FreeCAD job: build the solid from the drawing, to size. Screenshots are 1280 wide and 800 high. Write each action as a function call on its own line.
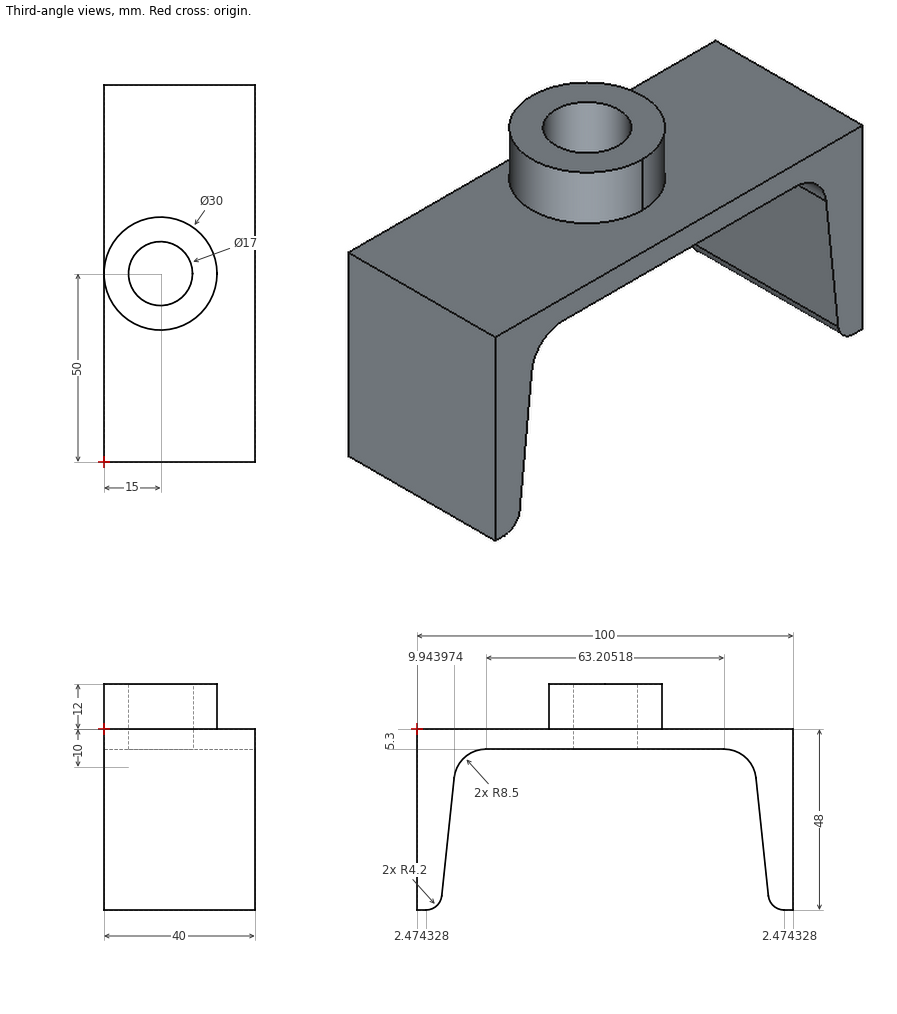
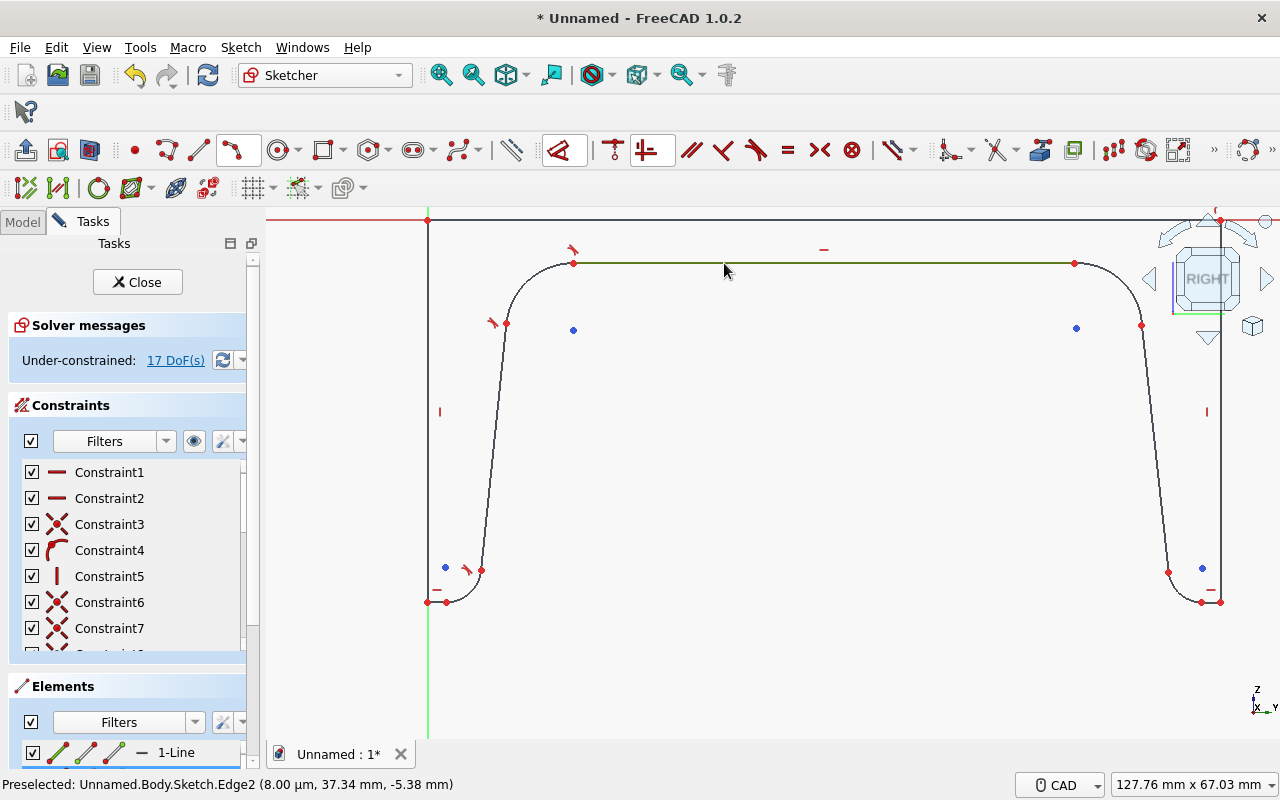
click(1104, 269)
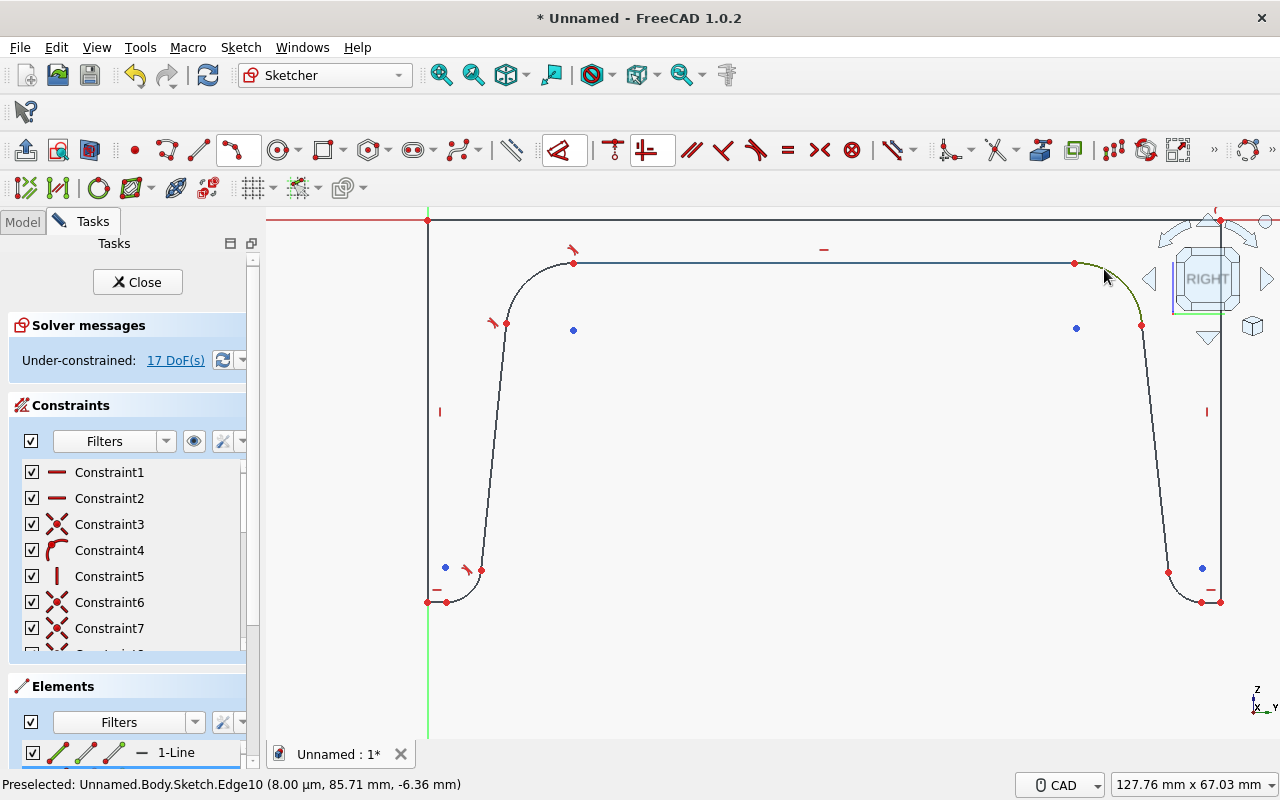
click(756, 150)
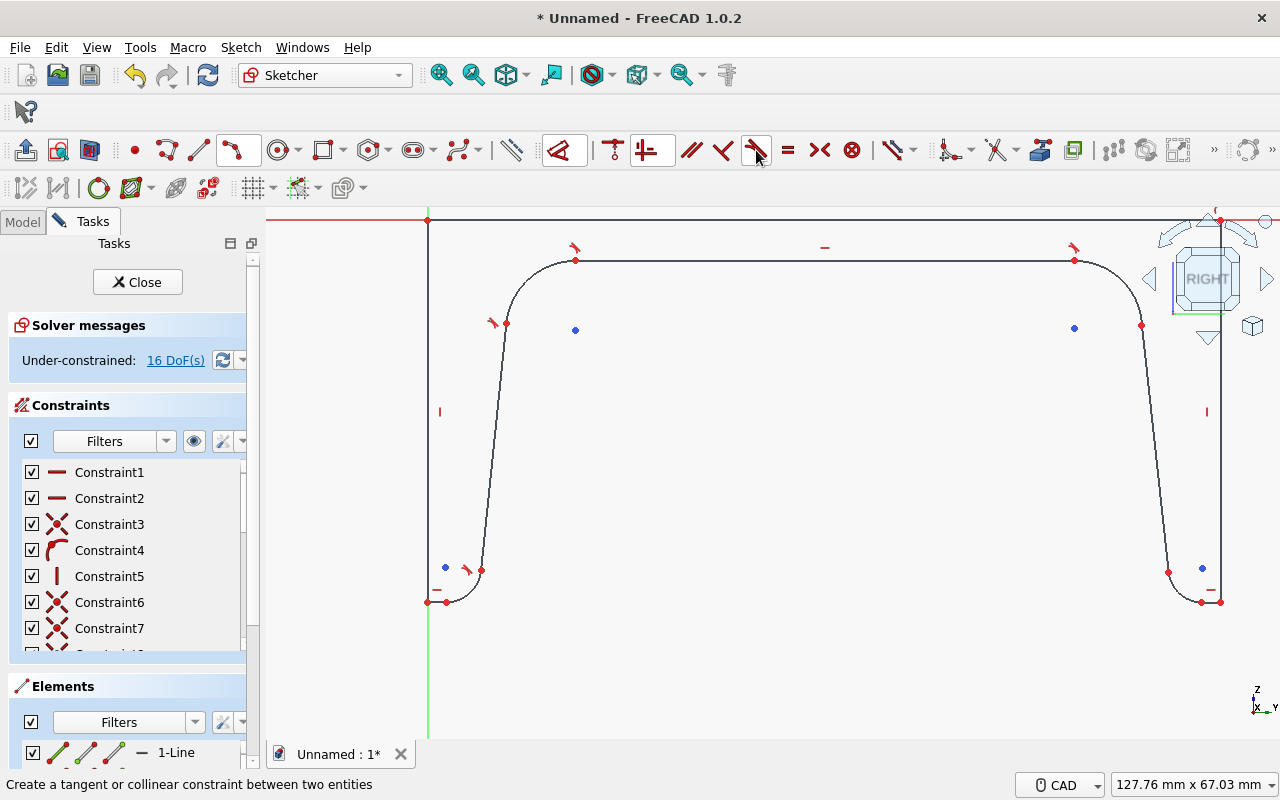
scroll(461, 599, down, 2)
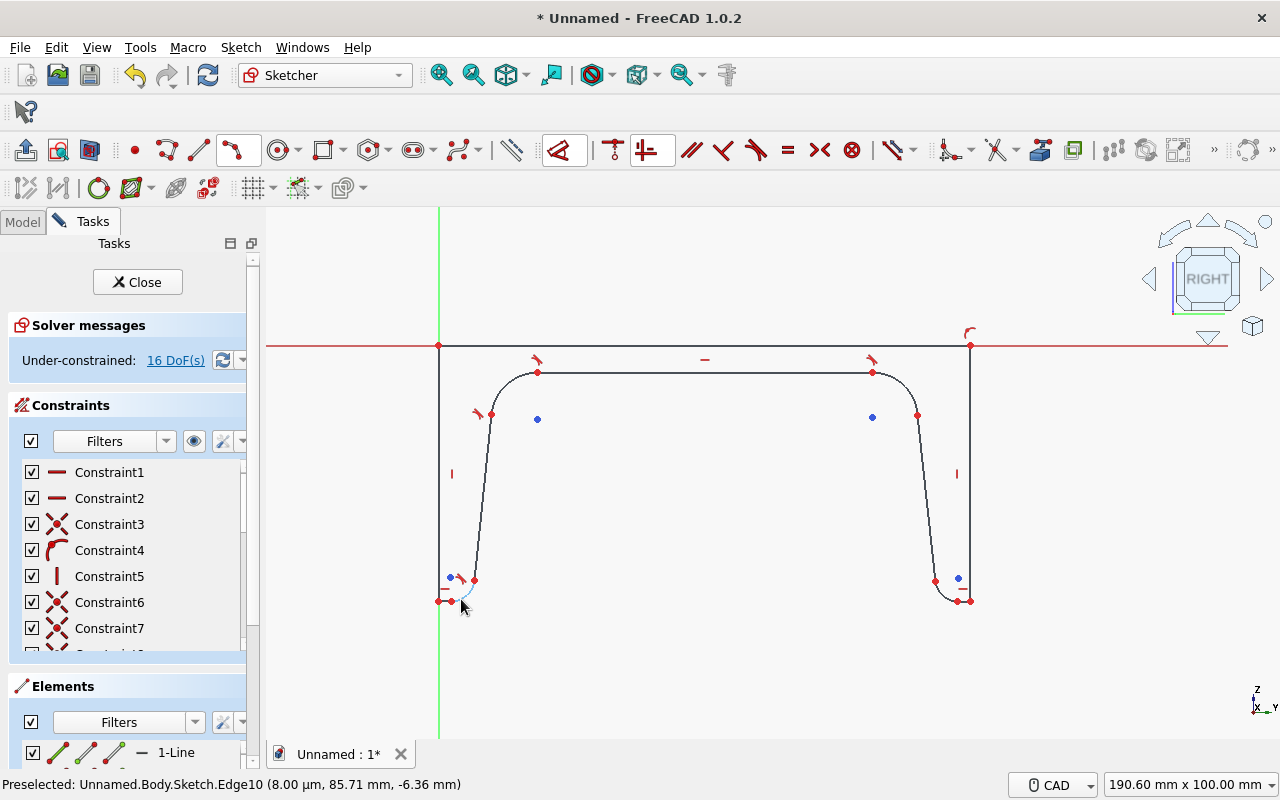
click(923, 465)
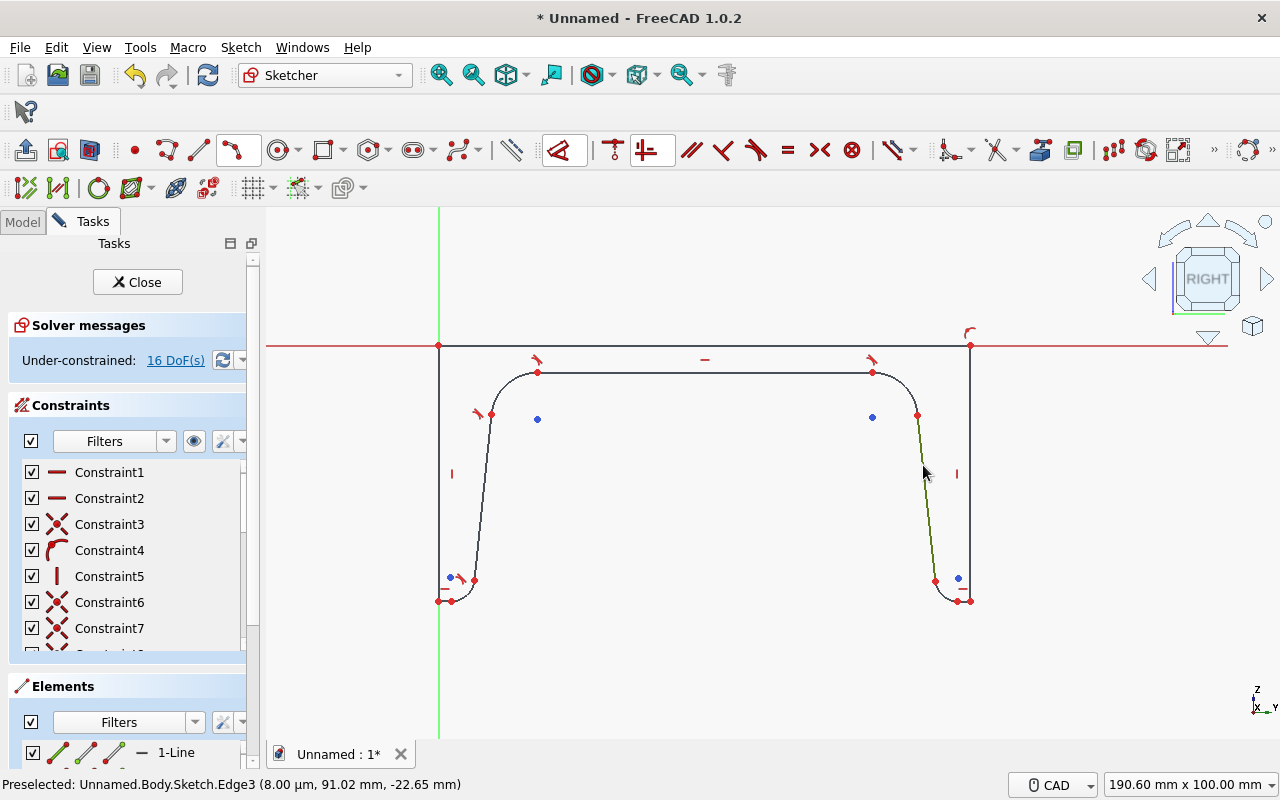
click(912, 396)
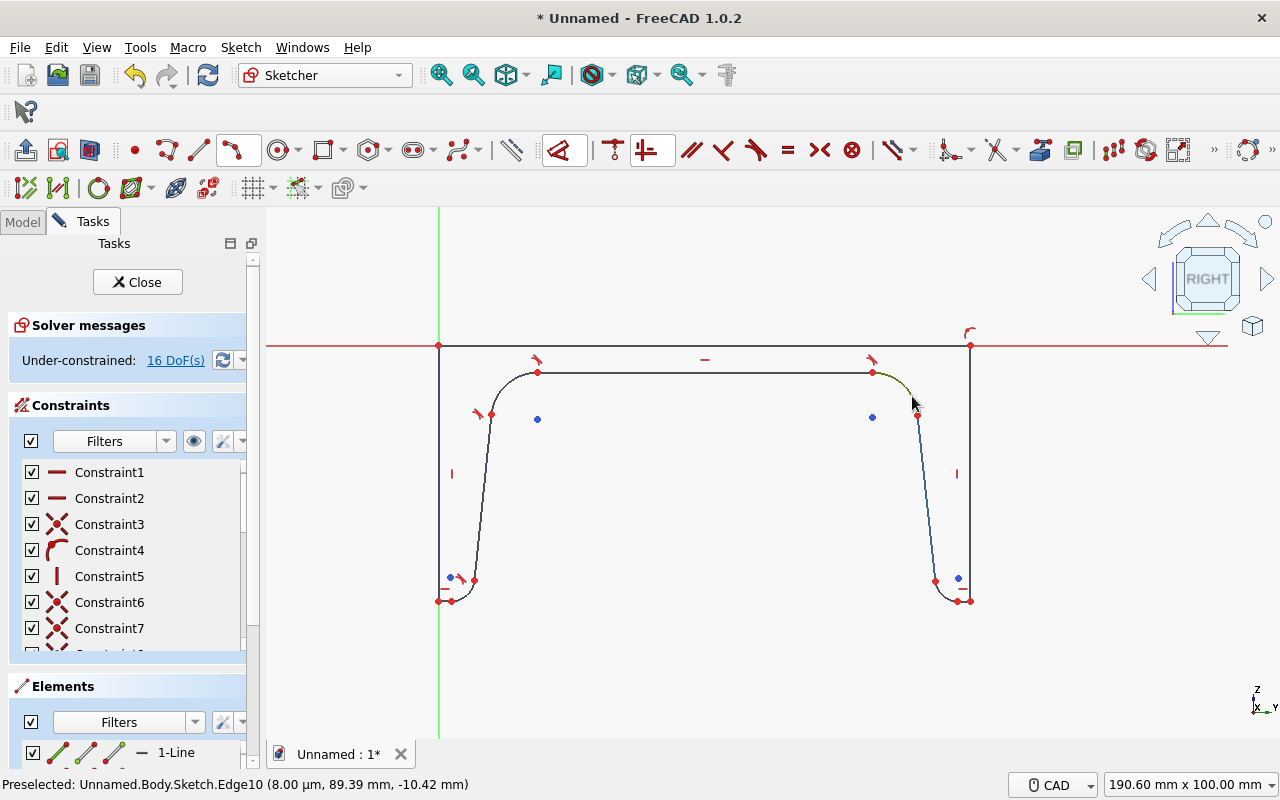
click(756, 150)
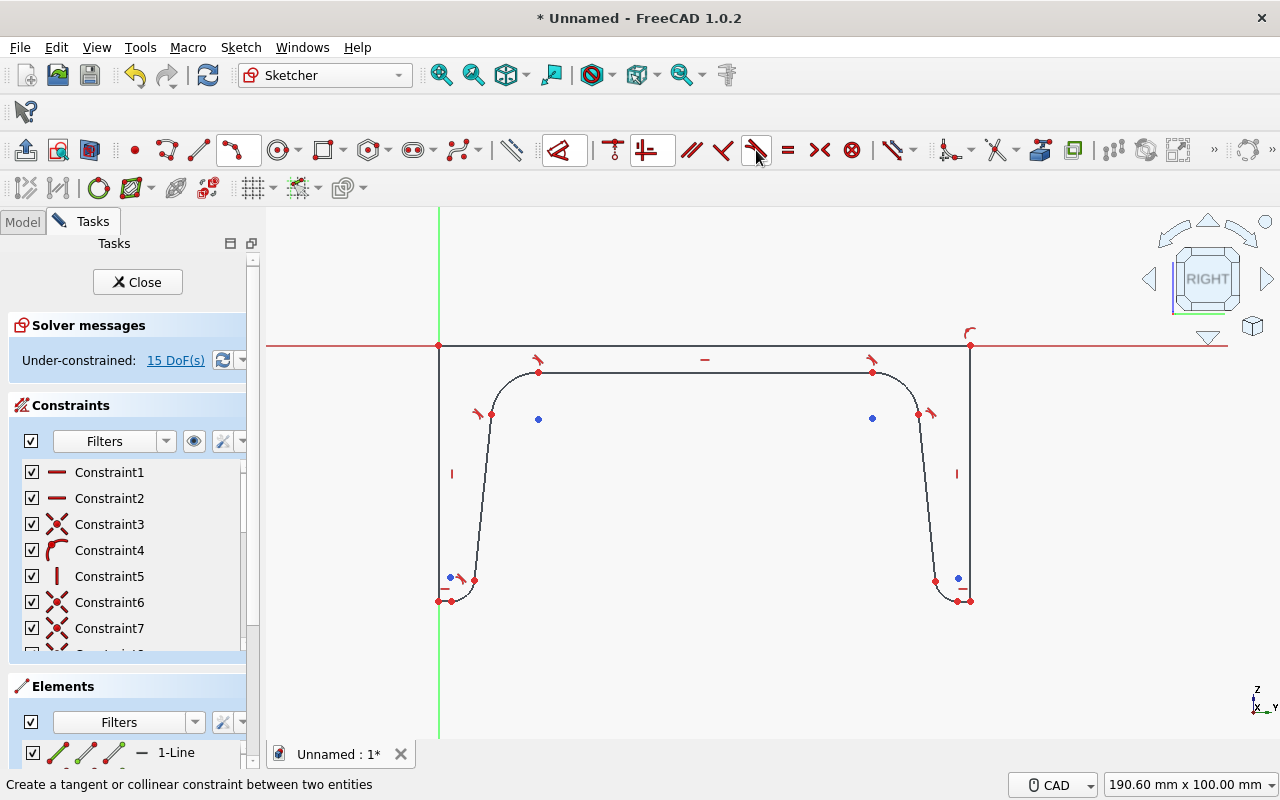
click(924, 465)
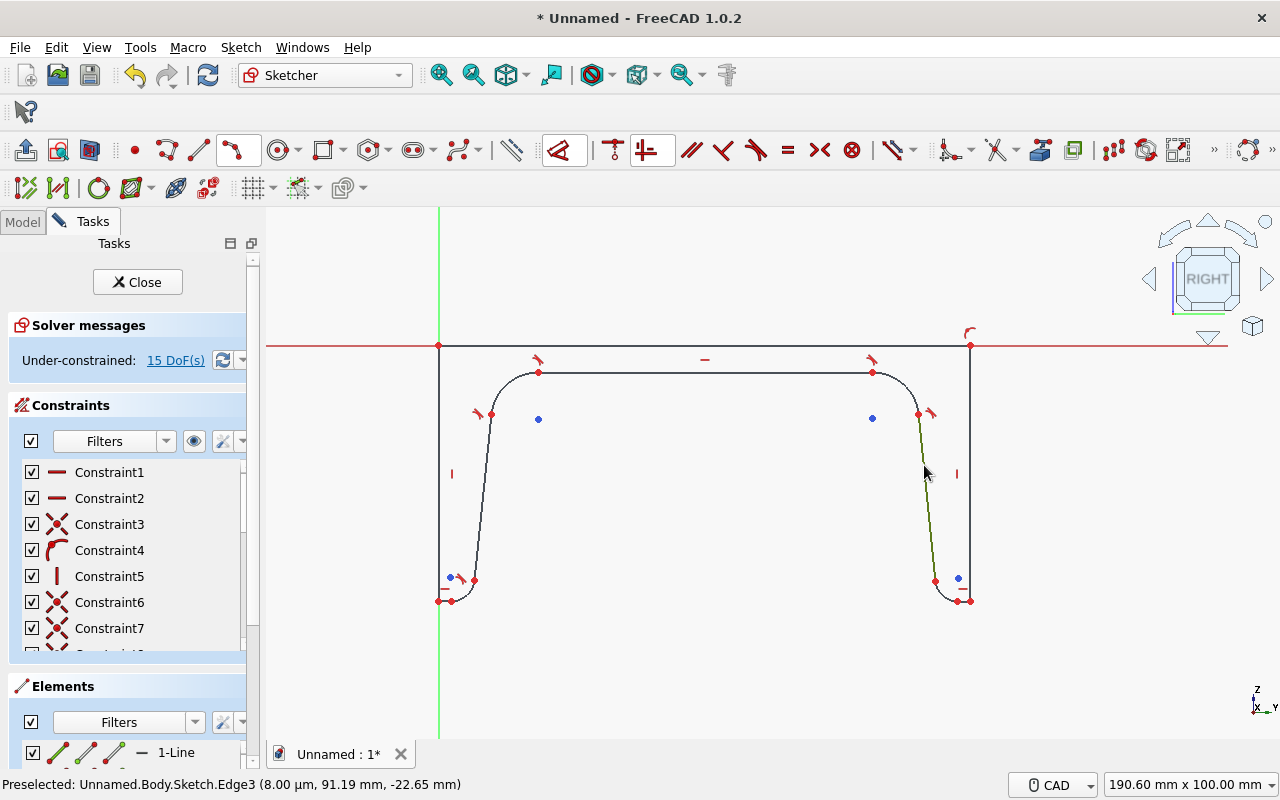
scroll(939, 591, up, 2)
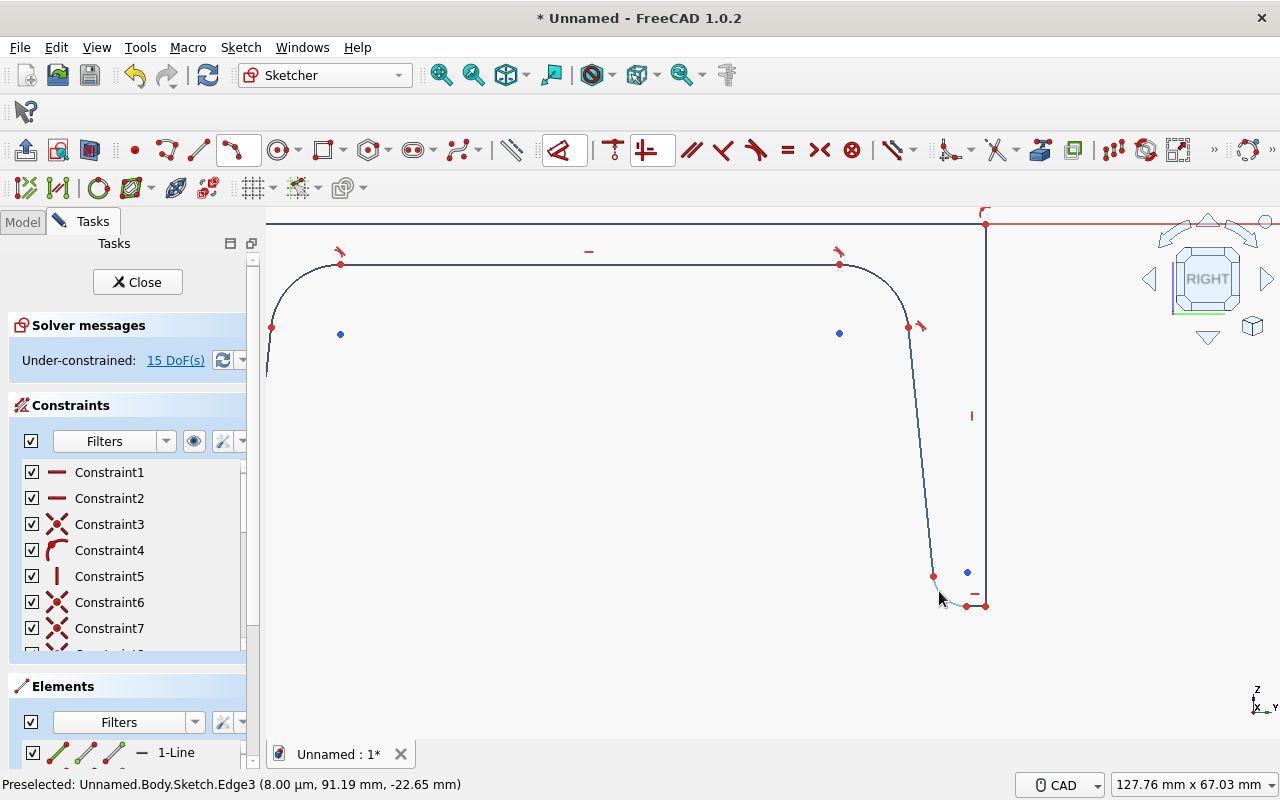
click(938, 590)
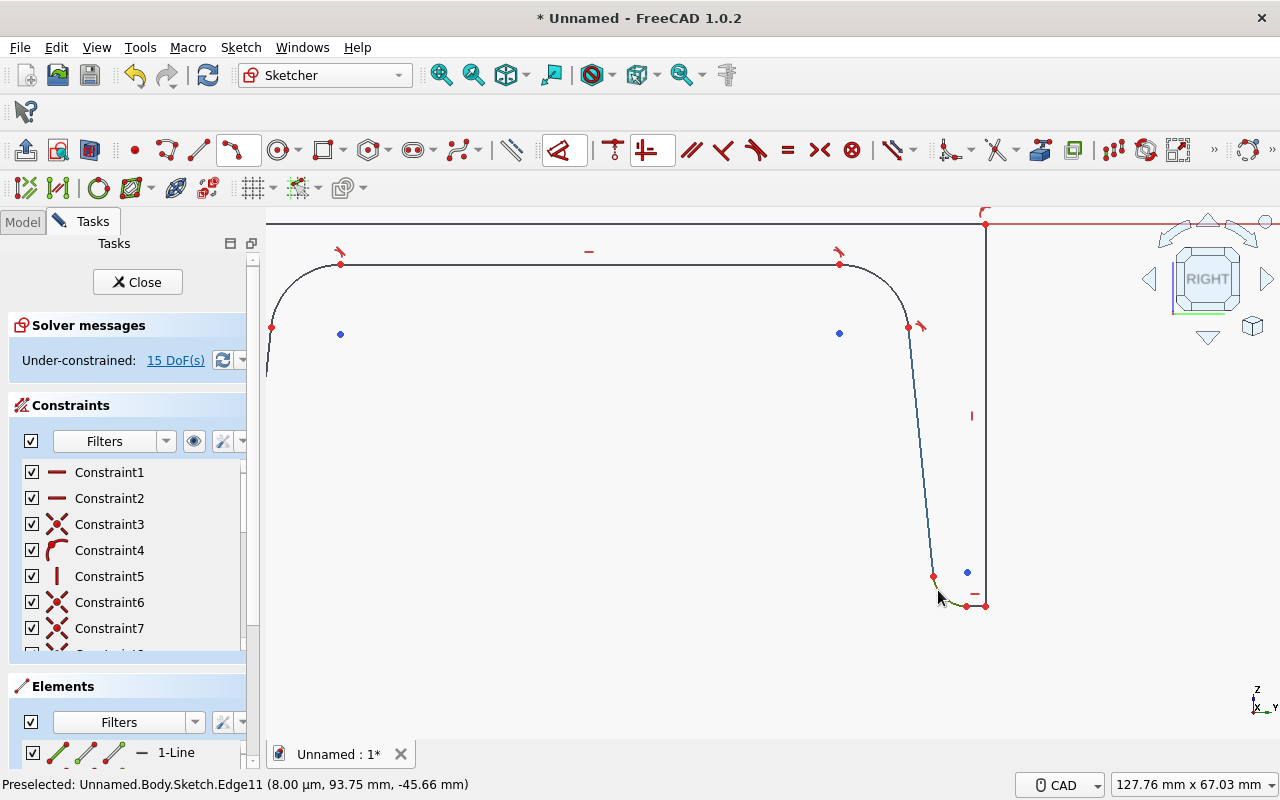
click(756, 150)